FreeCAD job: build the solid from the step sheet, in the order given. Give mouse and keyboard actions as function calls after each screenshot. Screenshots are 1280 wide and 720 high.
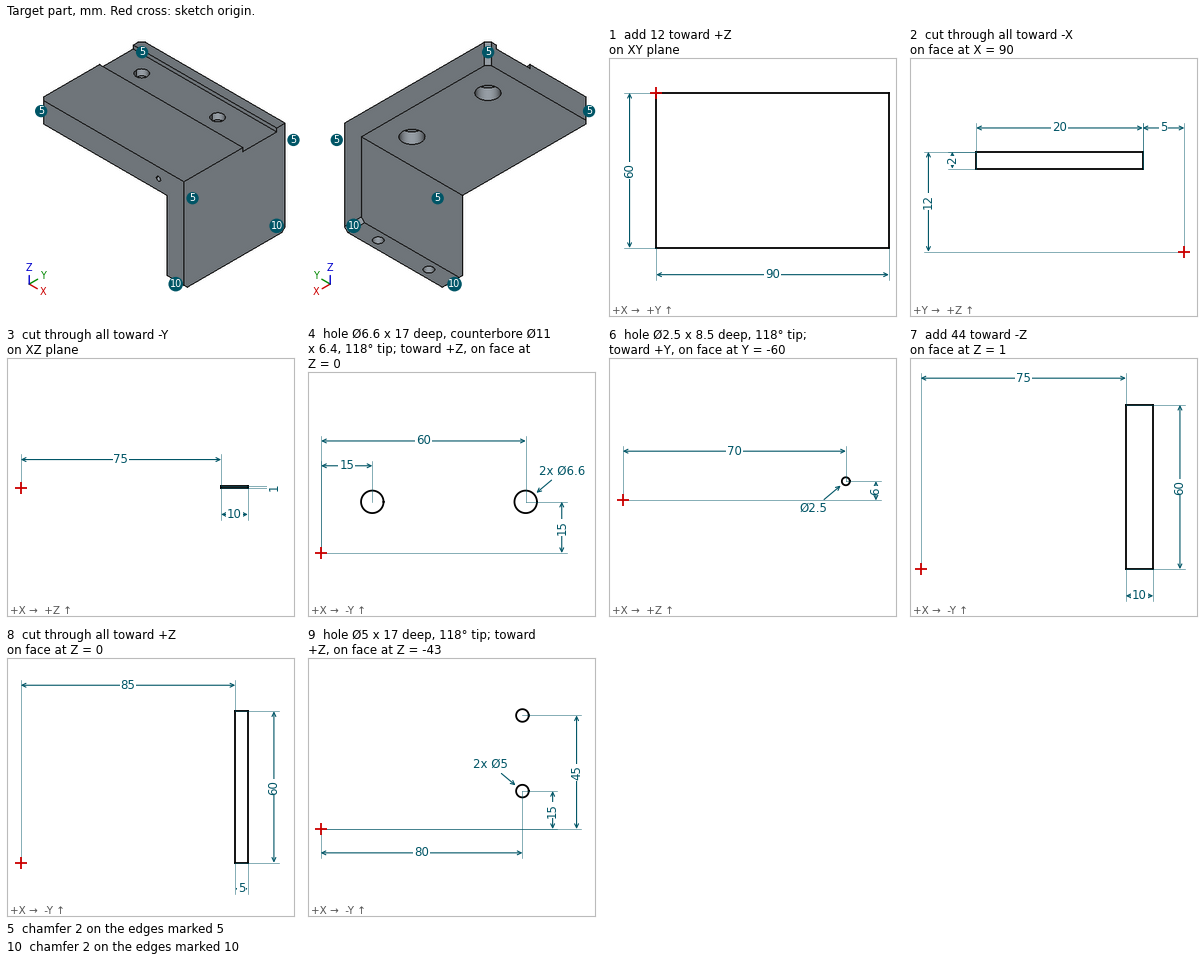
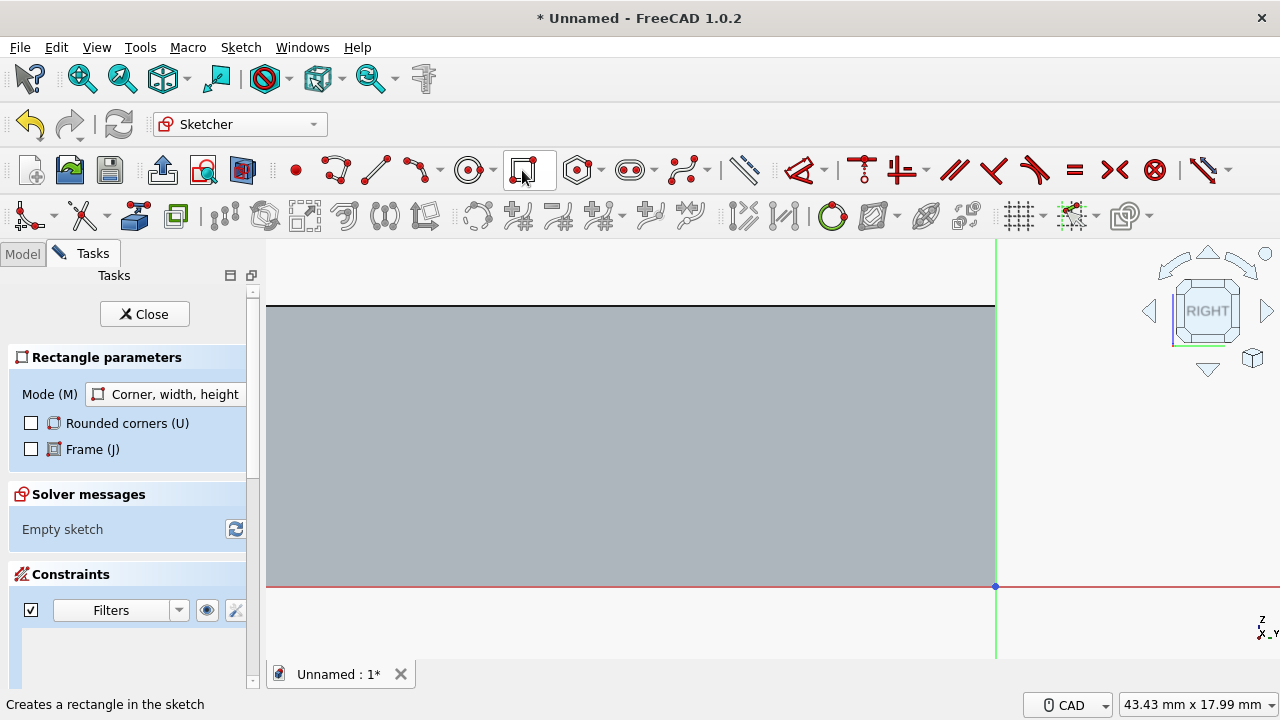
click(412, 306)
click(879, 353)
key(Escape)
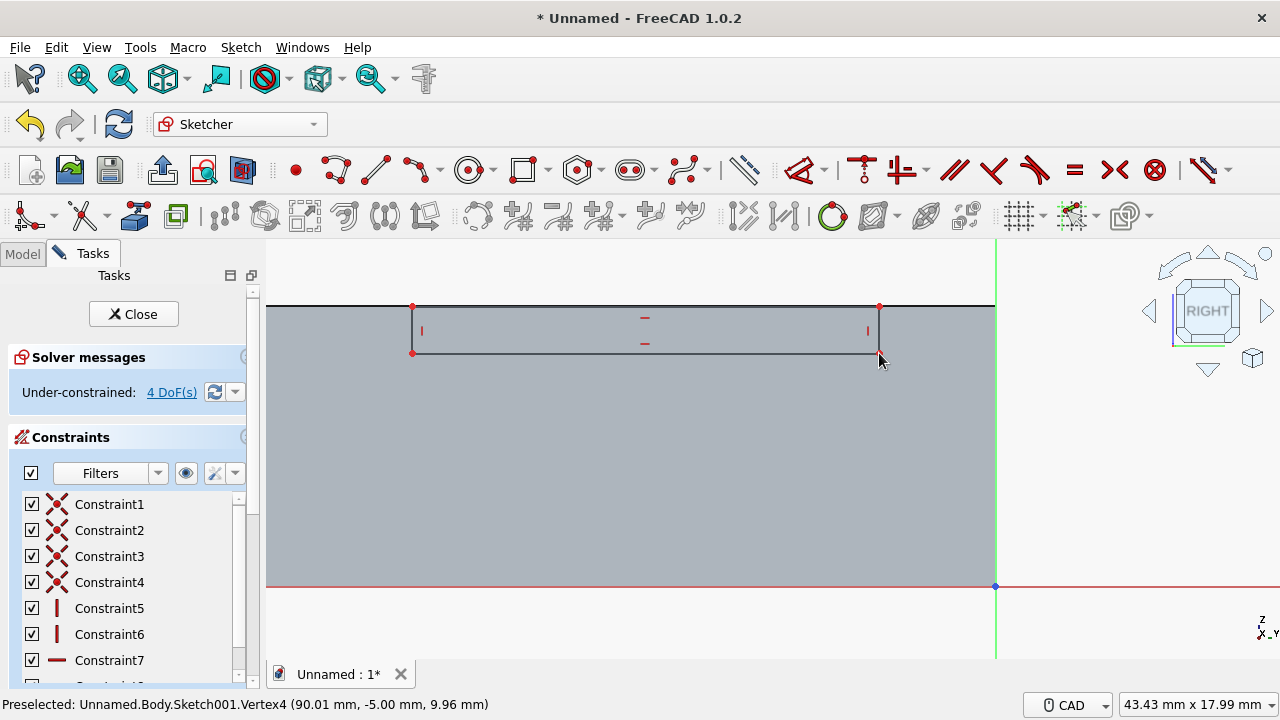
click(800, 170)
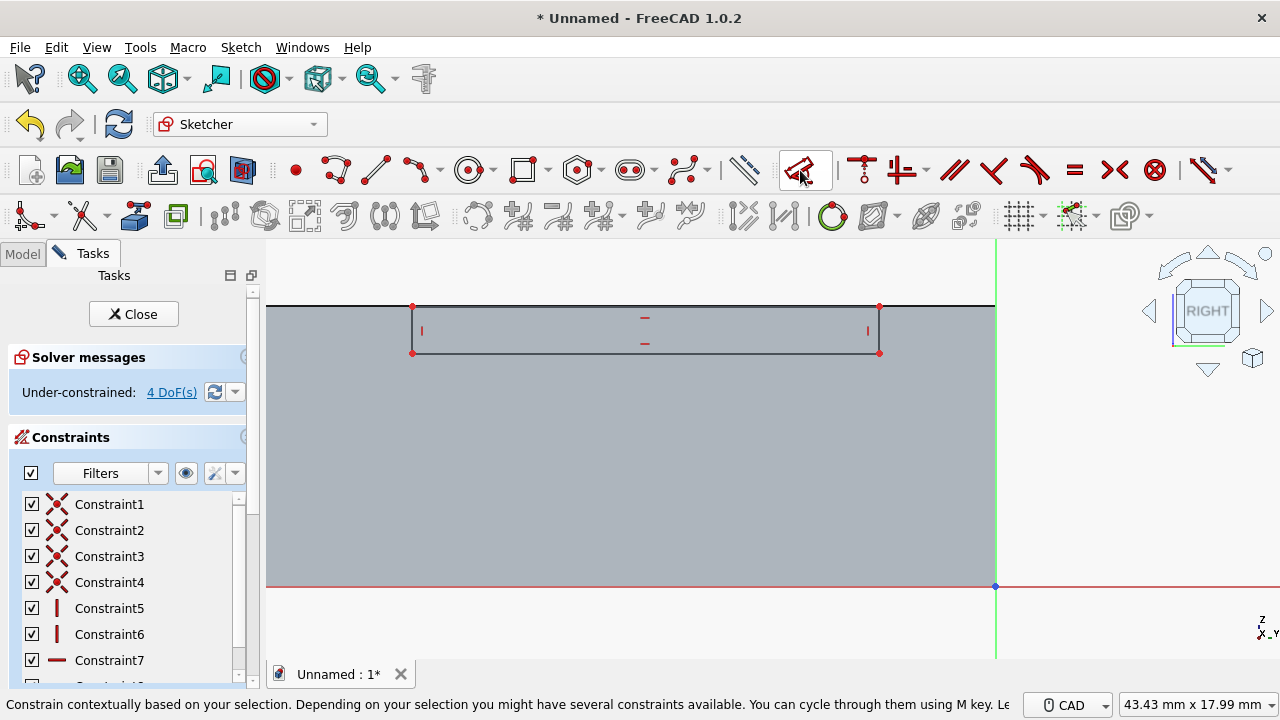
click(412, 321)
click(378, 331)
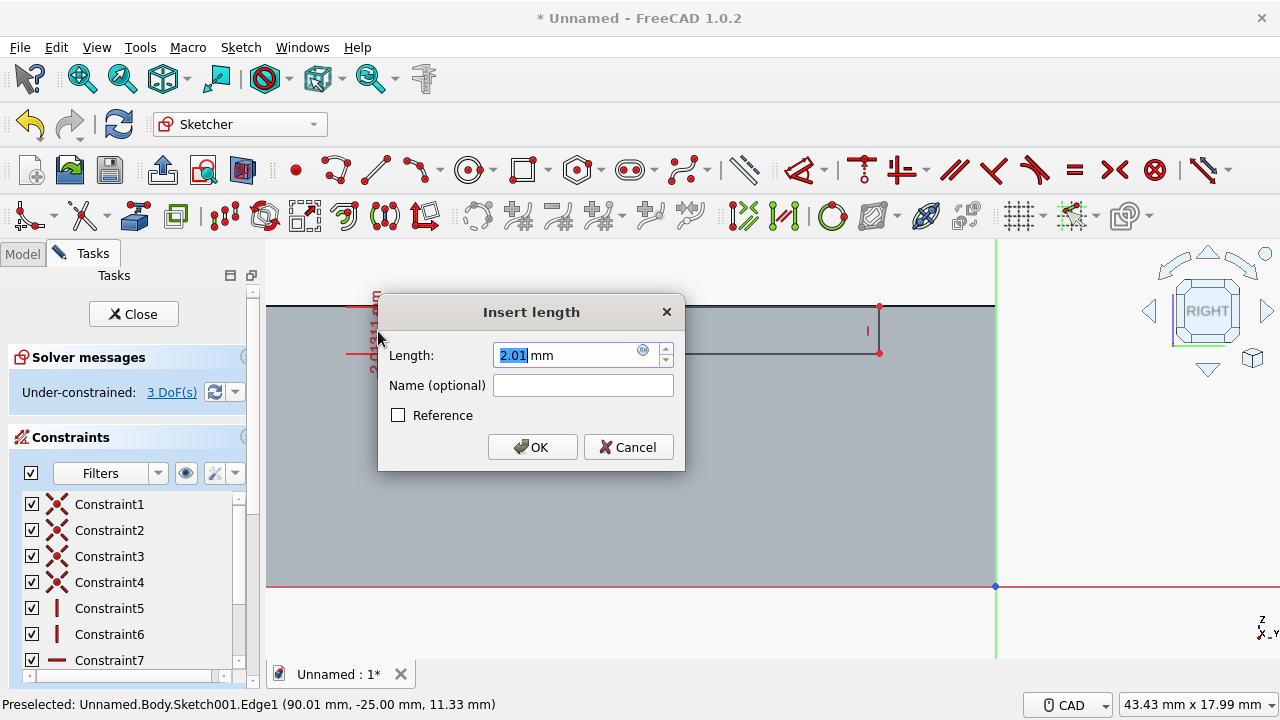
text(2)
key(Return)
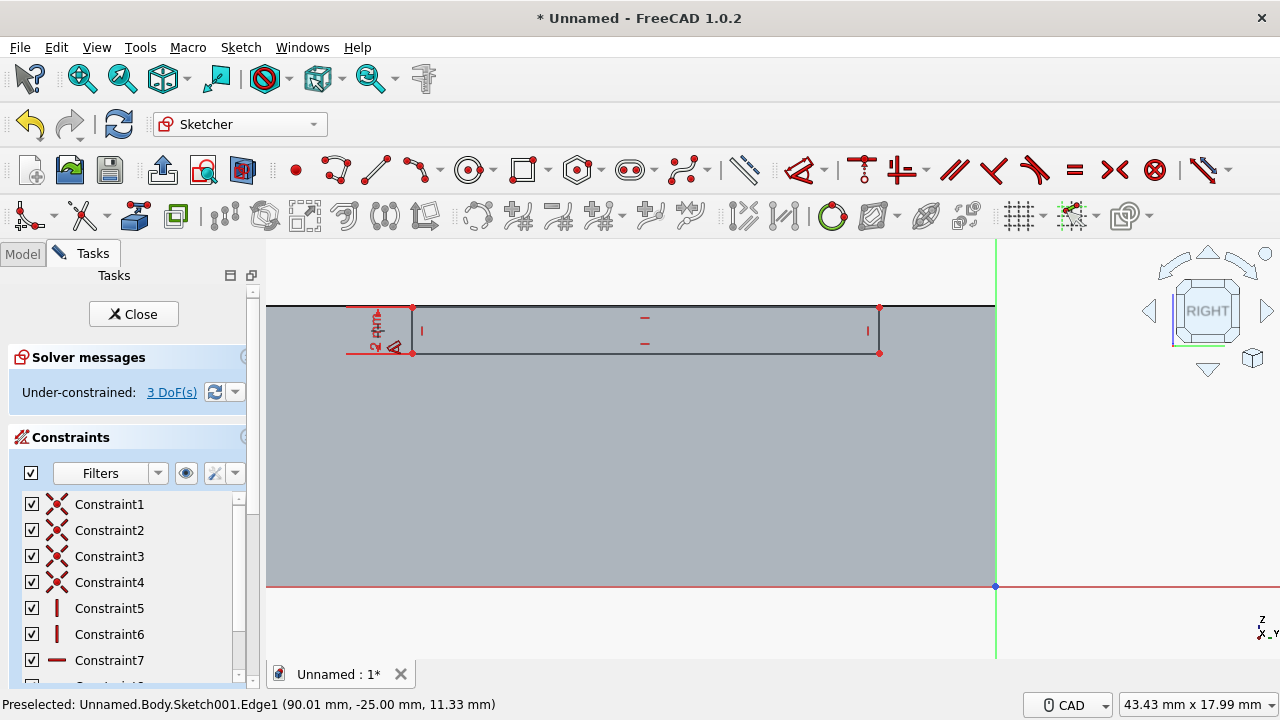
click(552, 354)
click(645, 388)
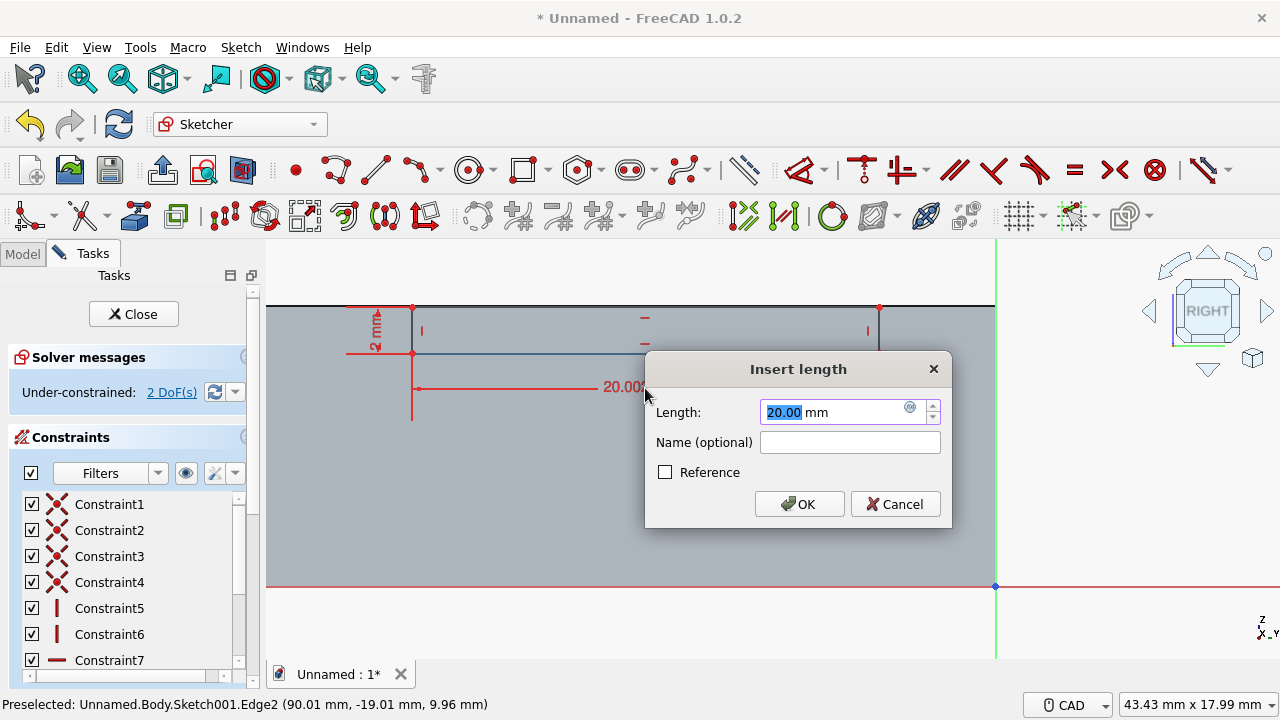
text(20)
key(Return)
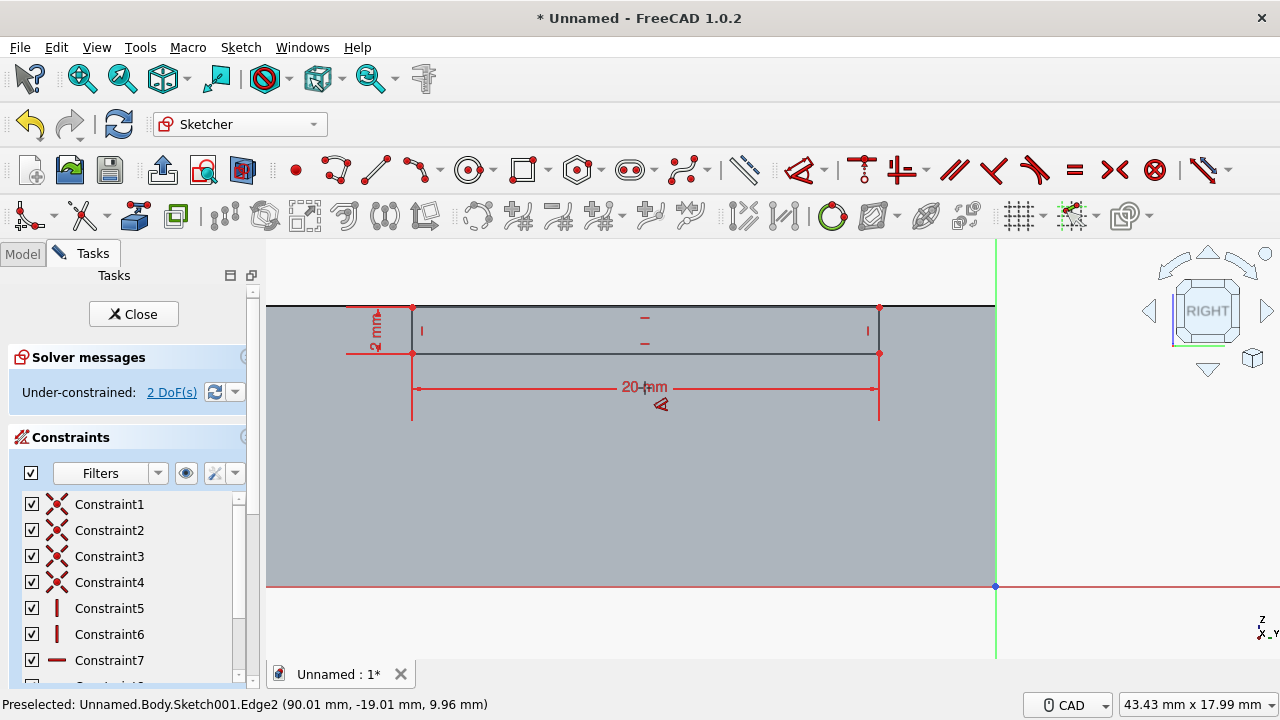
click(879, 354)
click(937, 621)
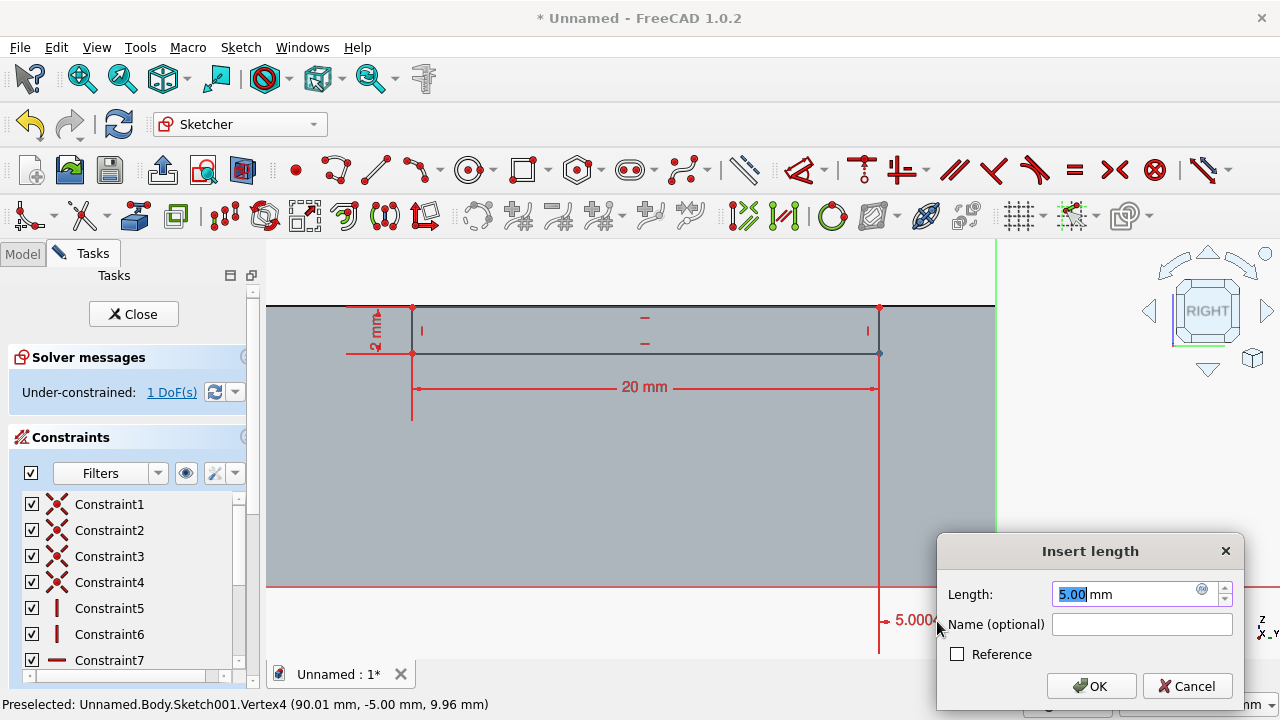
text(5)
key(Return)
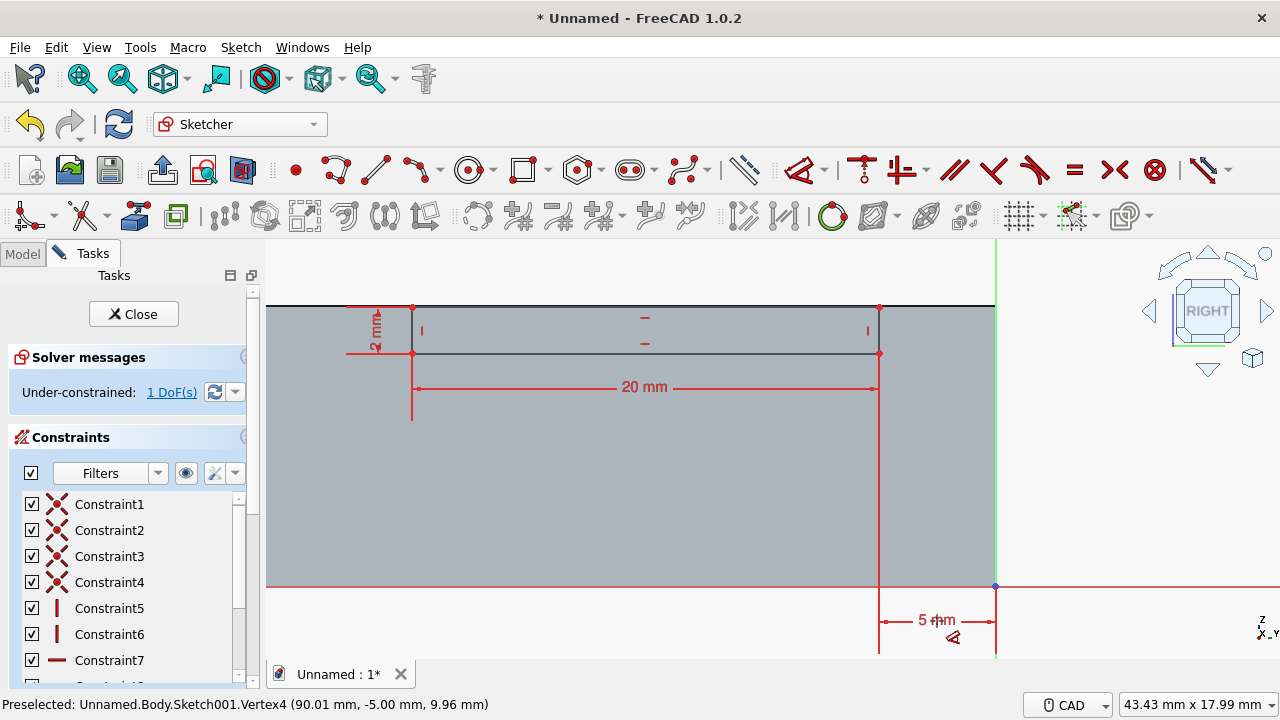
click(412, 307)
click(1030, 447)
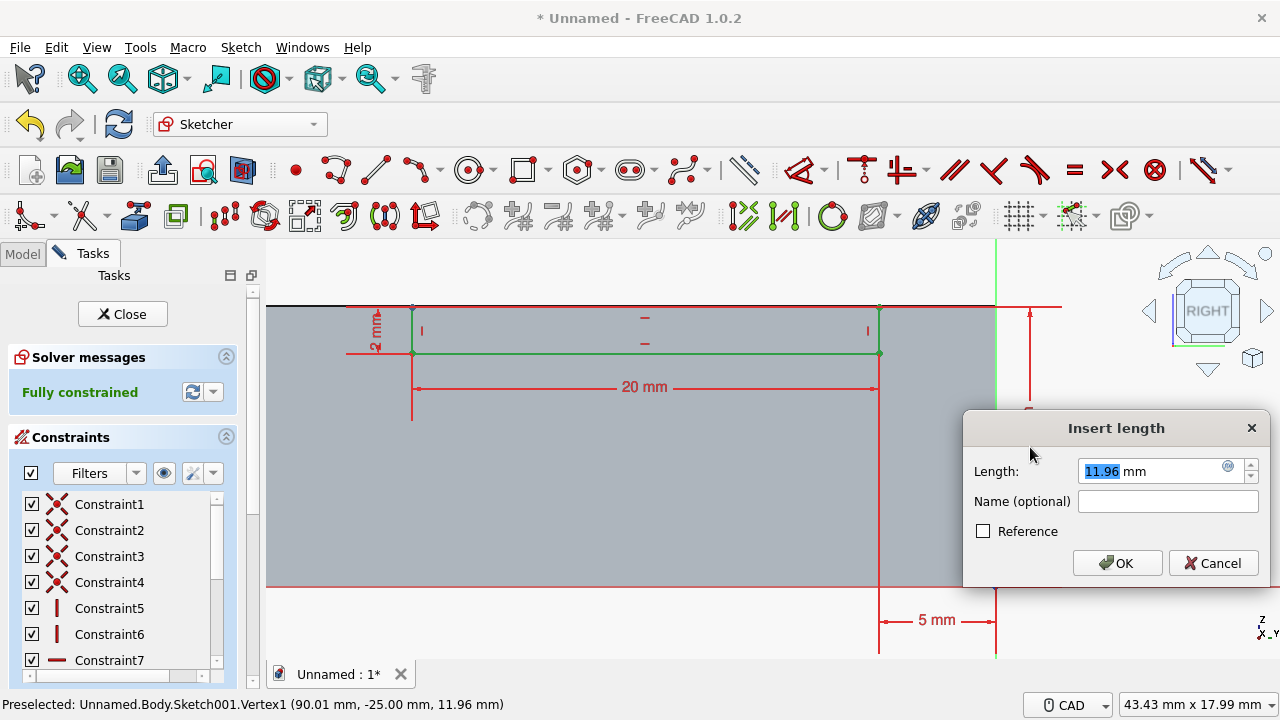
text(12)
key(Return)
key(Escape)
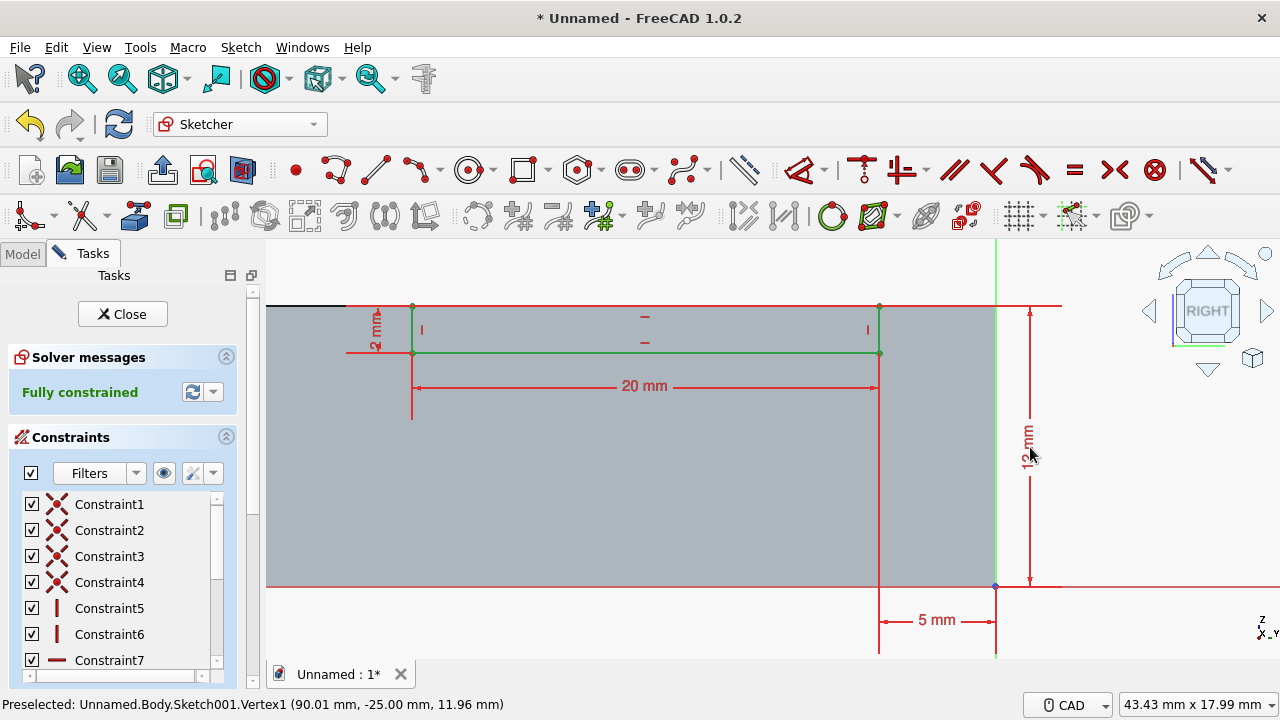
click(123, 314)